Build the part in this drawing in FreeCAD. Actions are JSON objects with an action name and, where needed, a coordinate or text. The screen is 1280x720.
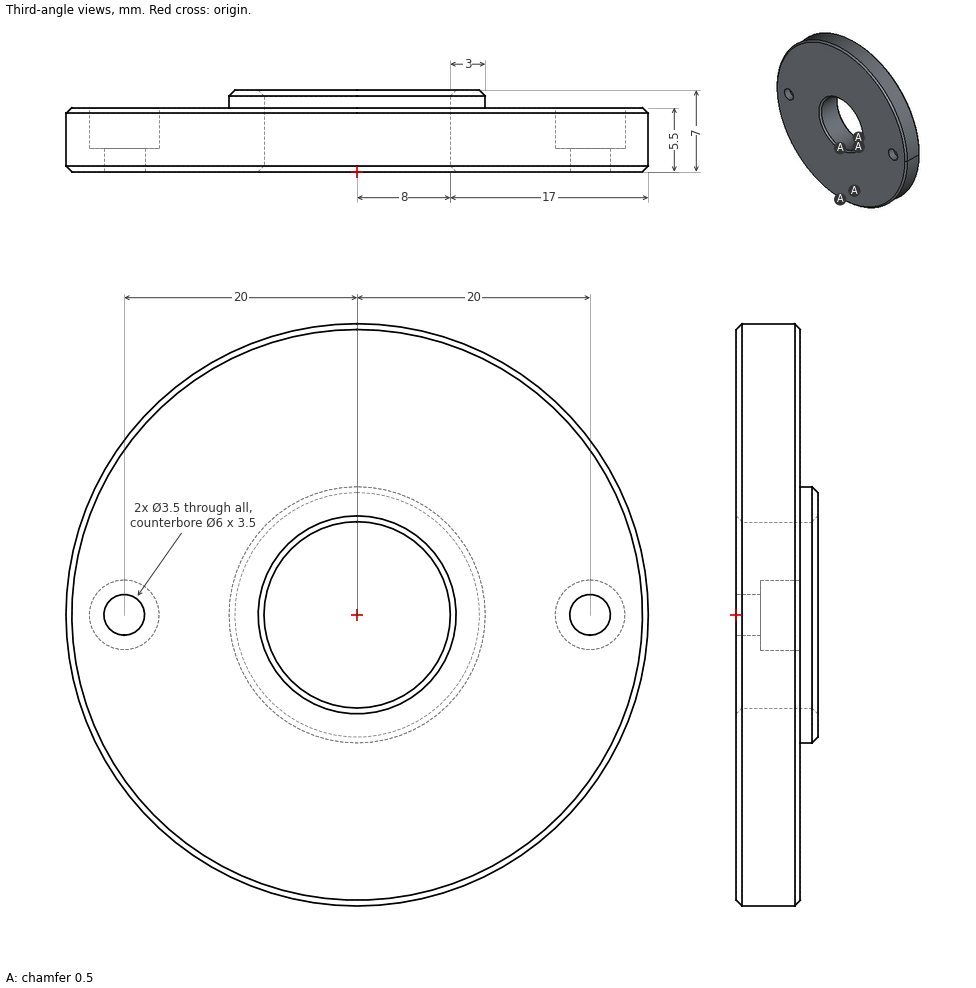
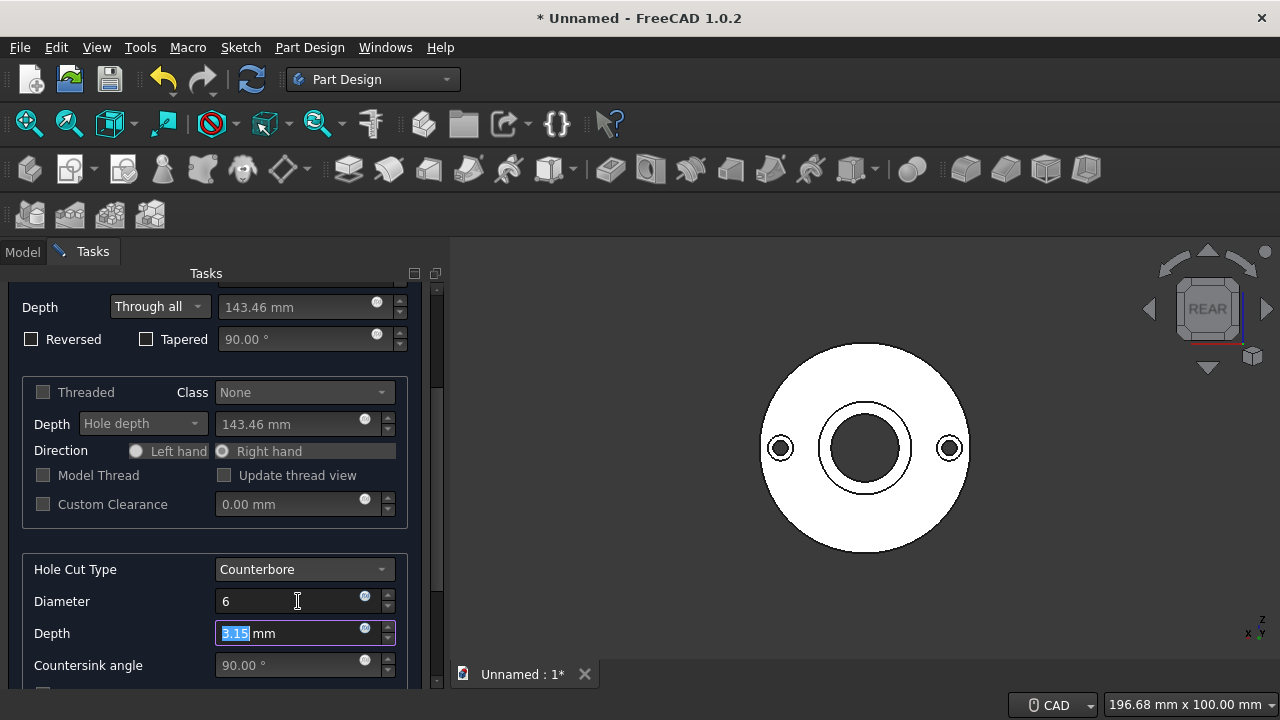
{"action": "type", "text": "3.5"}
{"action": "key", "text": "Tab"}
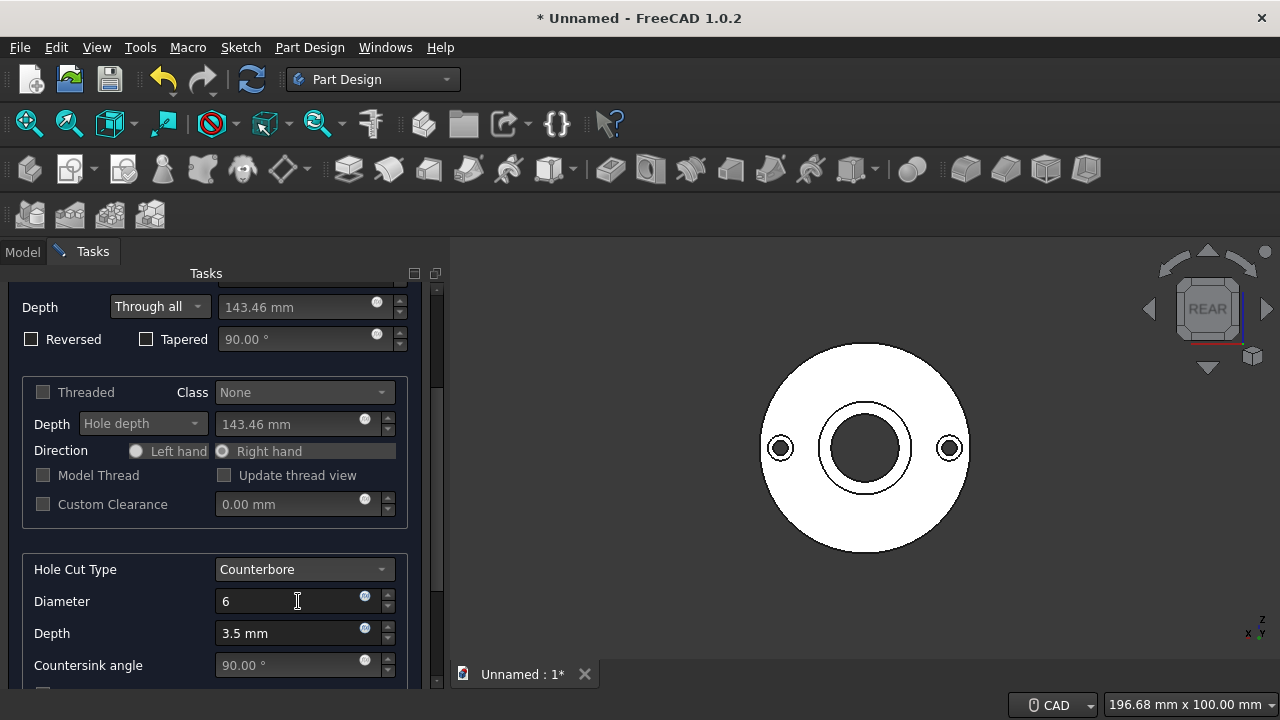
{"action": "scroll", "coordinate": [437, 486], "scroll_direction": "up", "scroll_amount": 4}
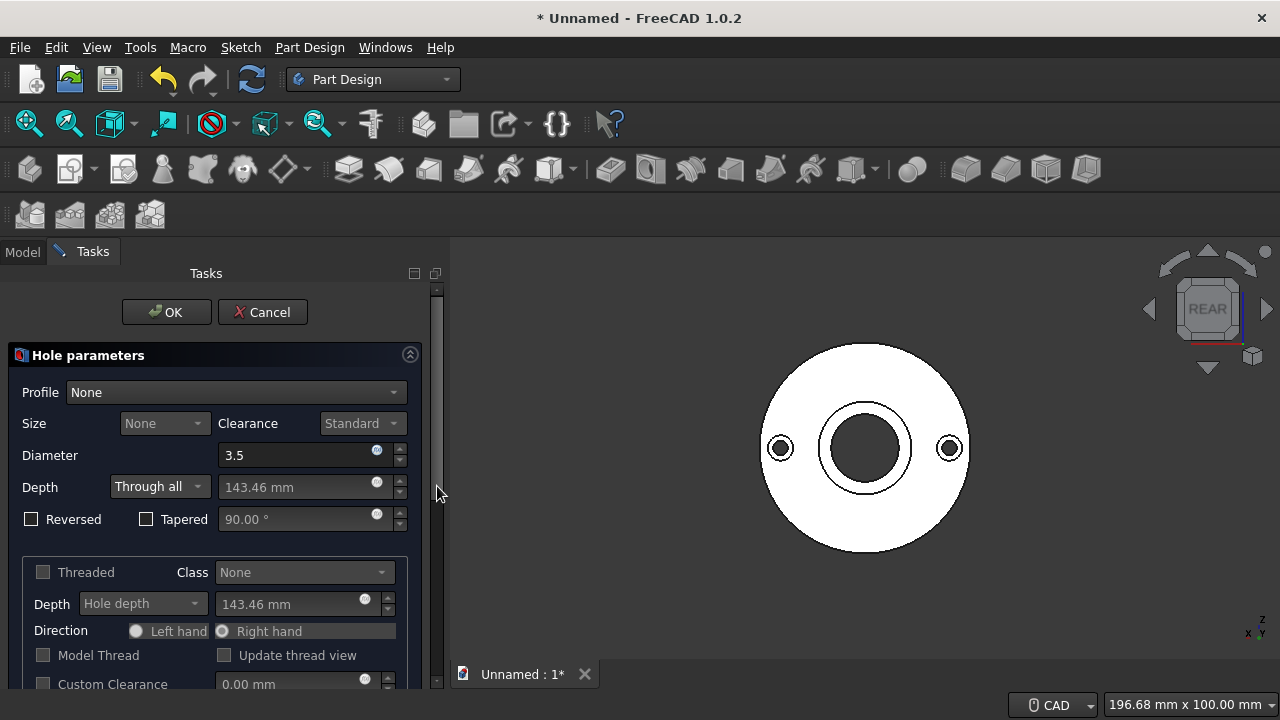
{"action": "left_click", "coordinate": [167, 312]}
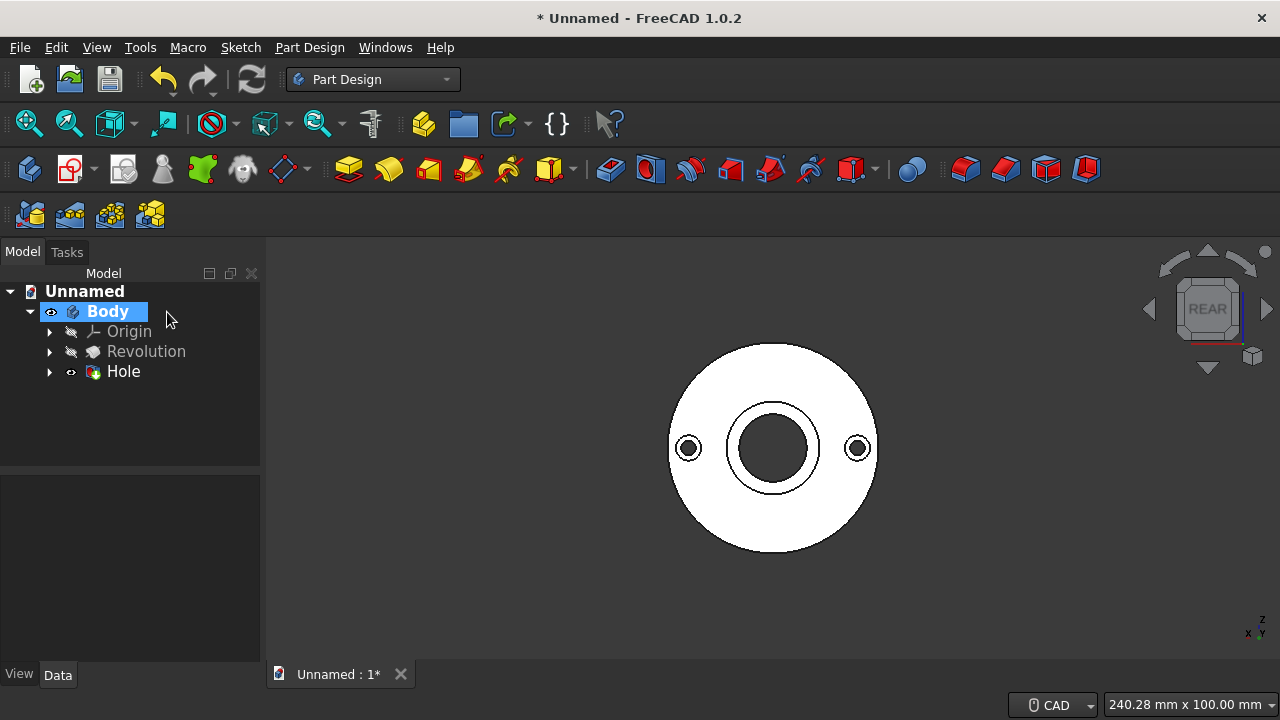
{"action": "left_click", "coordinate": [800, 427]}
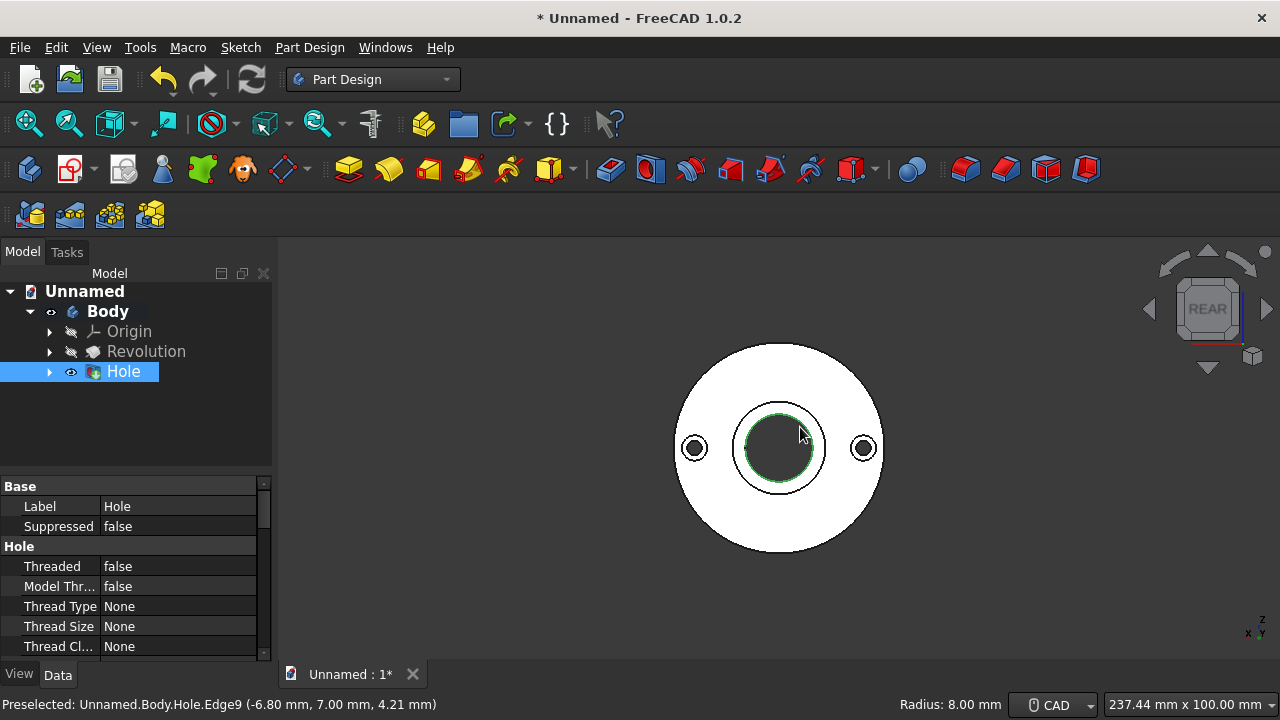
{"action": "left_click", "coordinate": [825, 447], "text": "ctrl"}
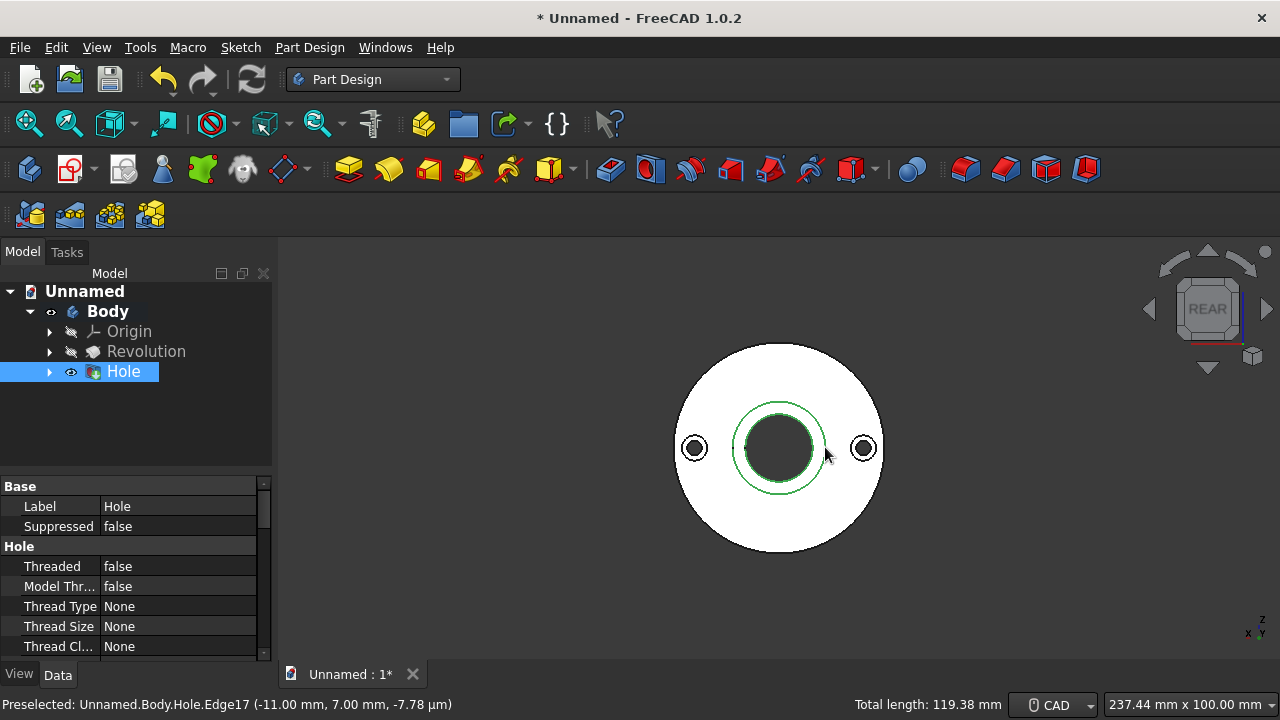
{"action": "left_click", "coordinate": [885, 447], "text": "ctrl"}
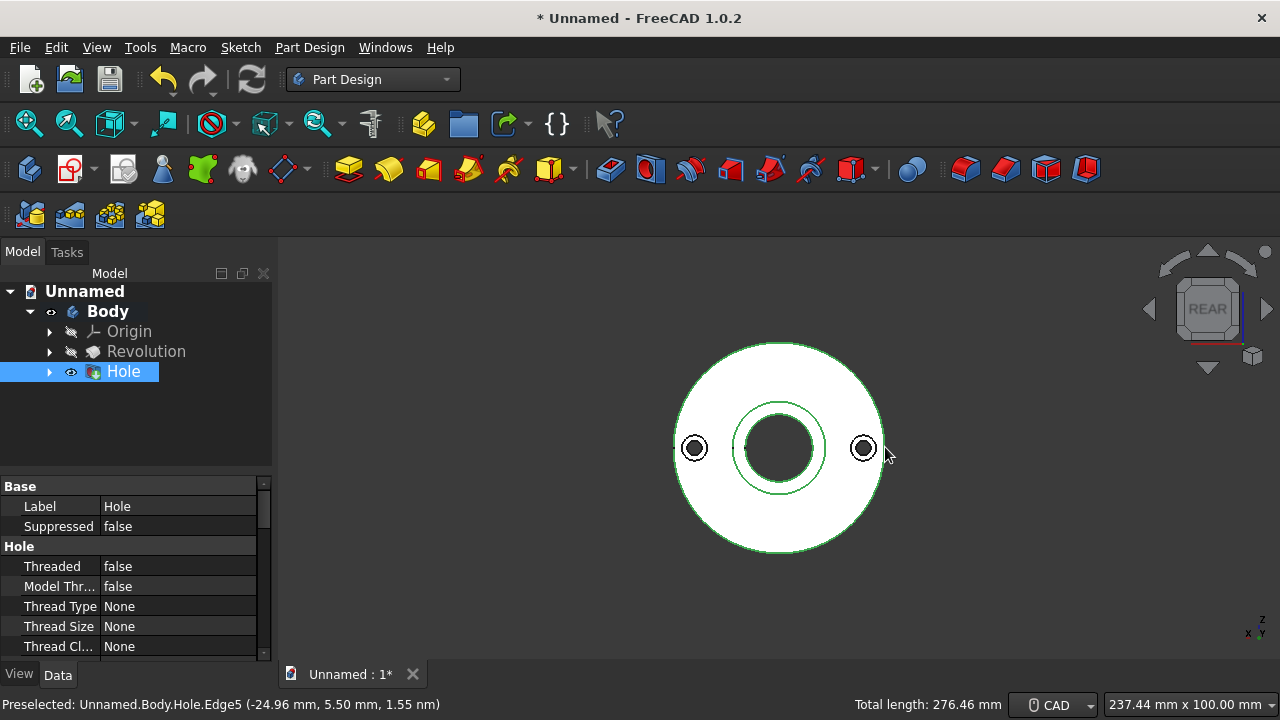
{"action": "key", "text": "0"}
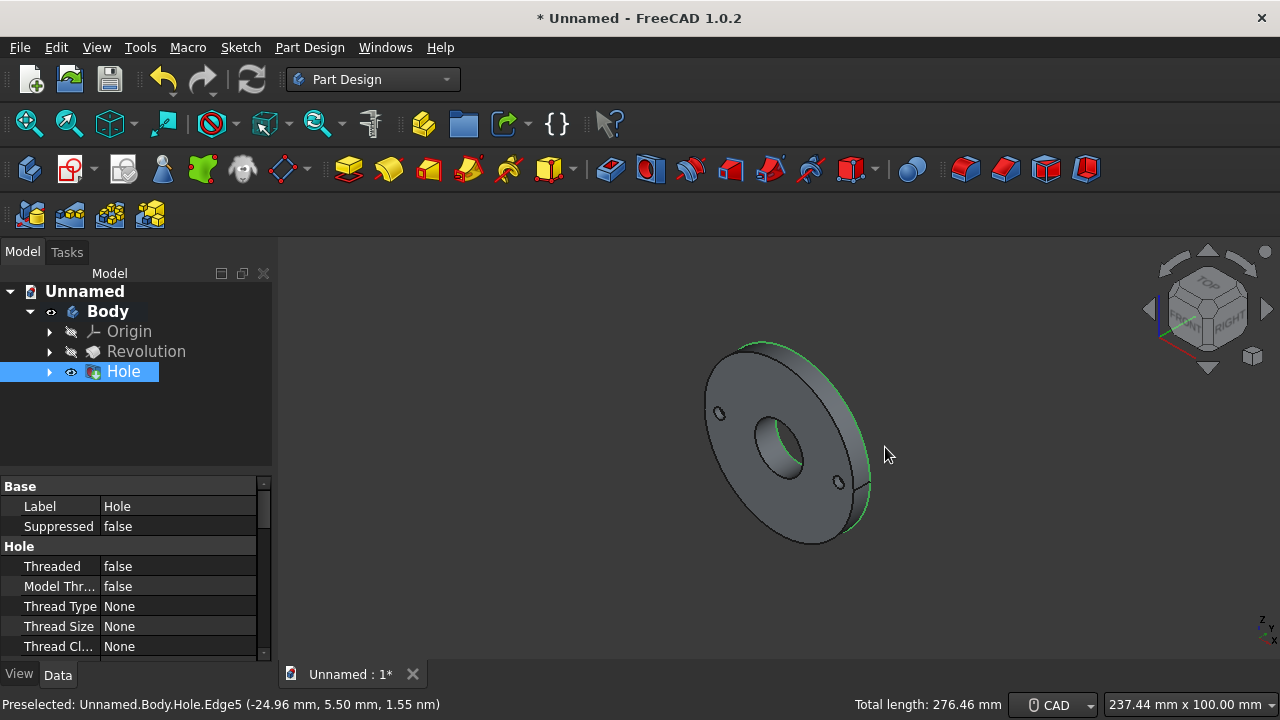
{"action": "left_click", "coordinate": [756, 352], "text": "ctrl"}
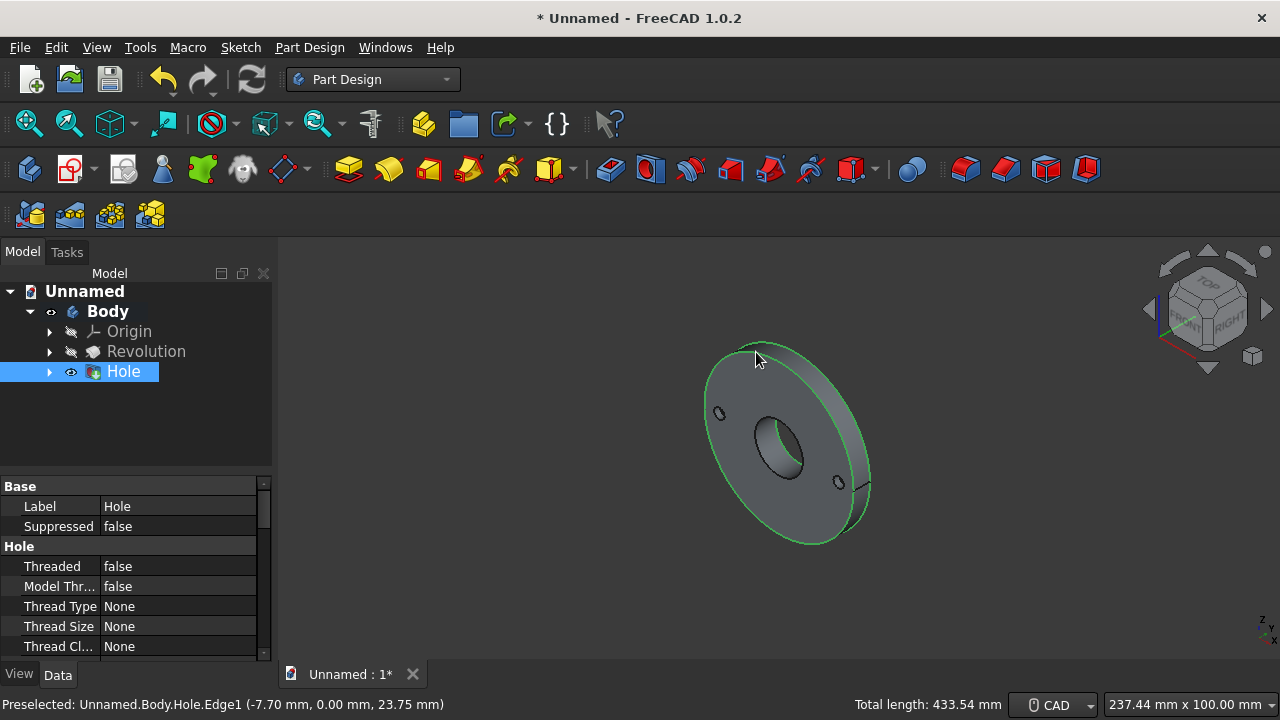
{"action": "left_click", "coordinate": [755, 433], "text": "ctrl"}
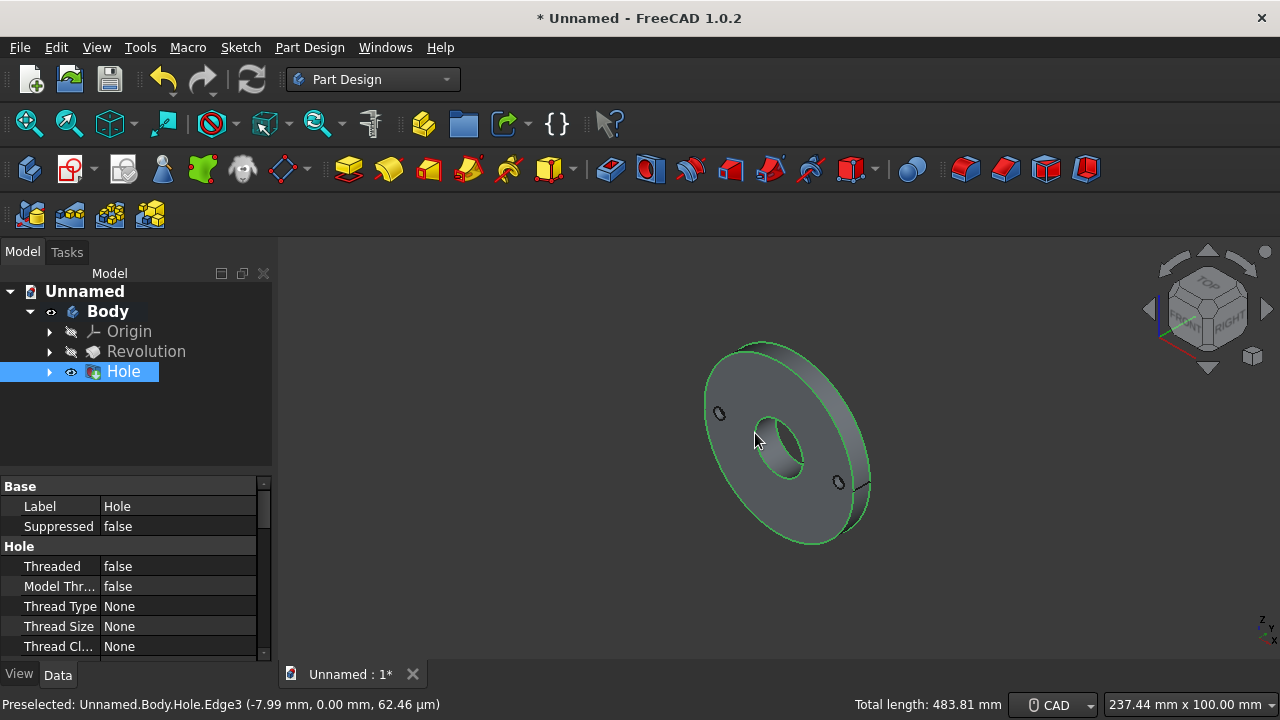
{"action": "left_click", "coordinate": [1006, 170]}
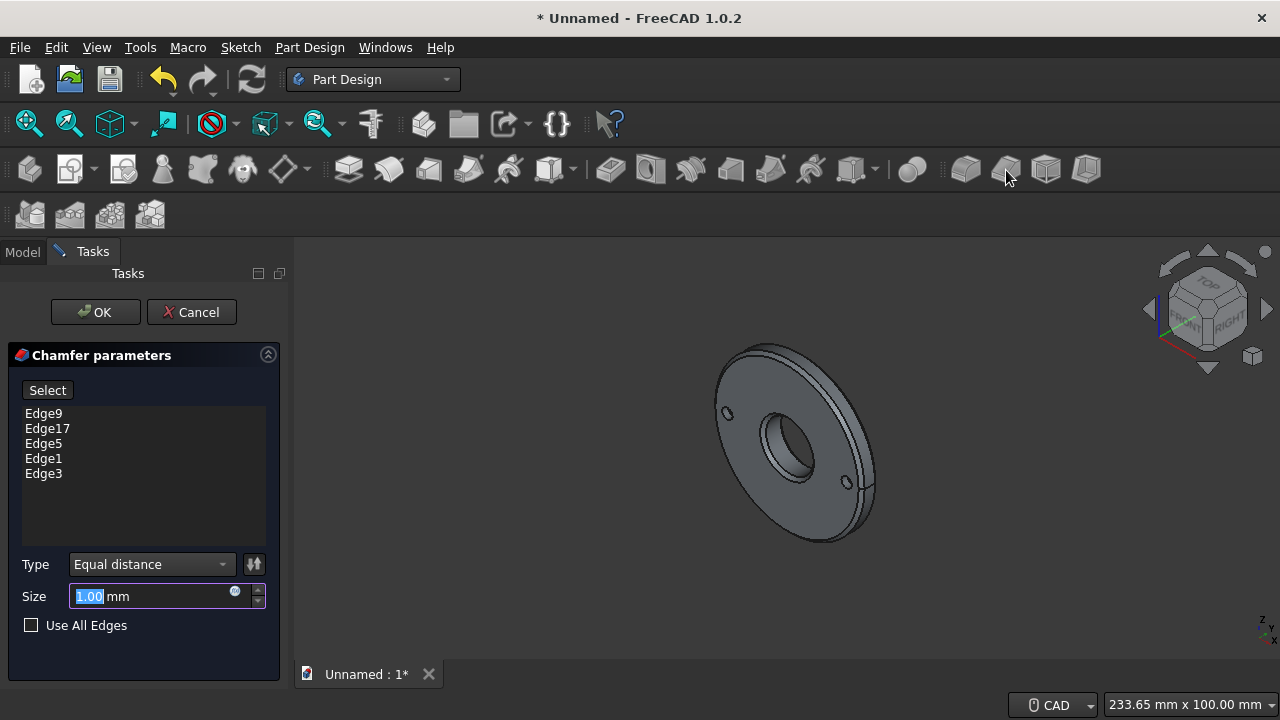
{"action": "type", "text": "0.5"}
{"action": "key", "text": "Tab"}